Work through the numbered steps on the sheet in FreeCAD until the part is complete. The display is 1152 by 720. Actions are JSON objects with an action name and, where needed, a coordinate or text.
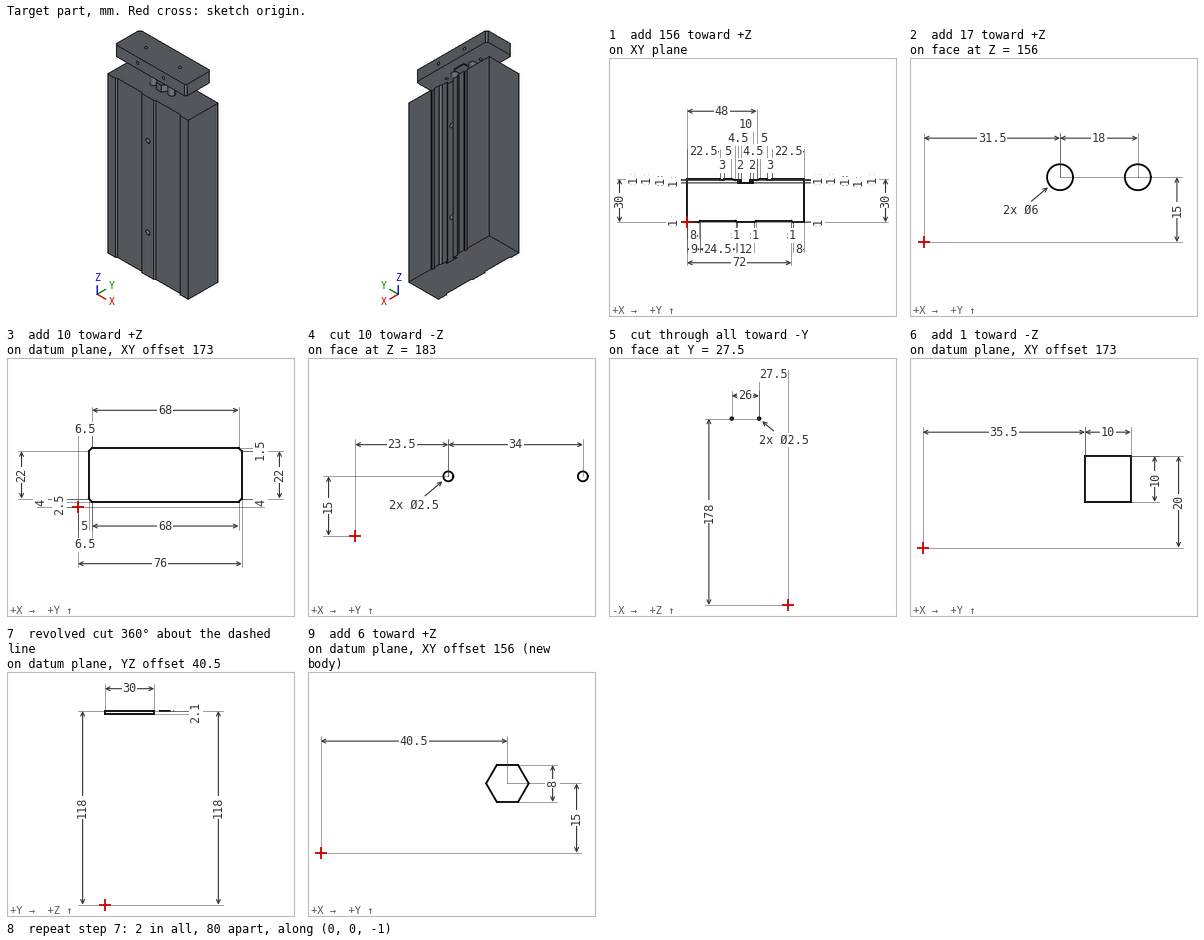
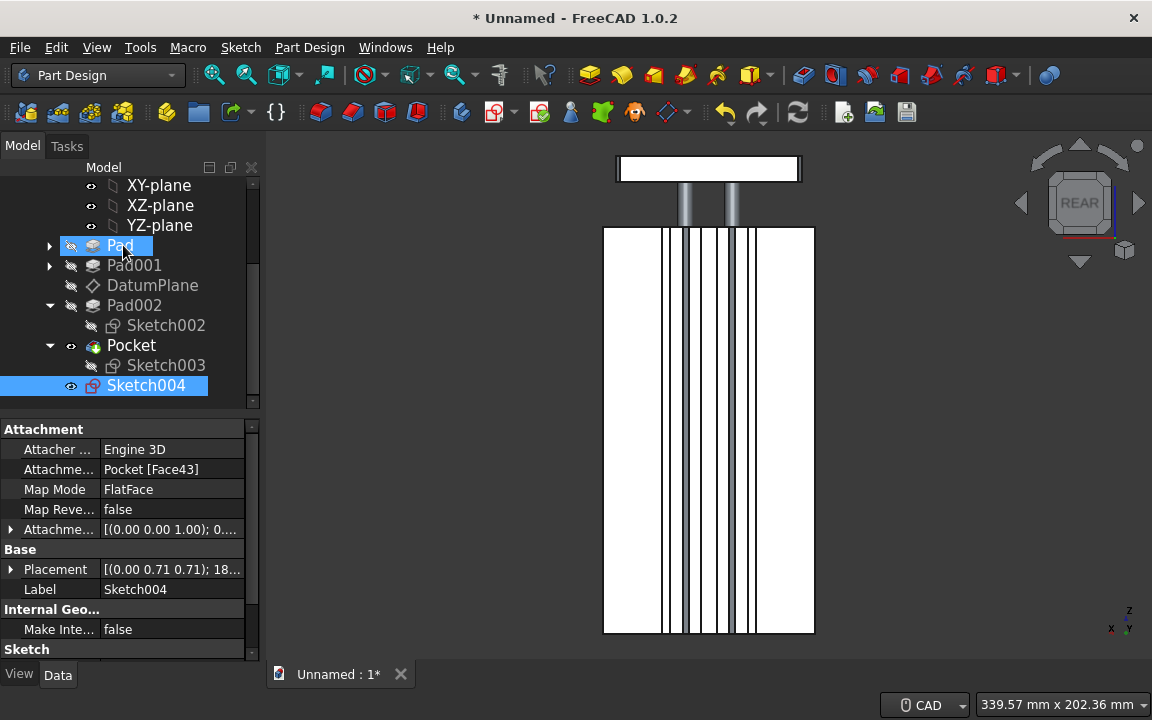
{"action": "left_click", "coordinate": [804, 76]}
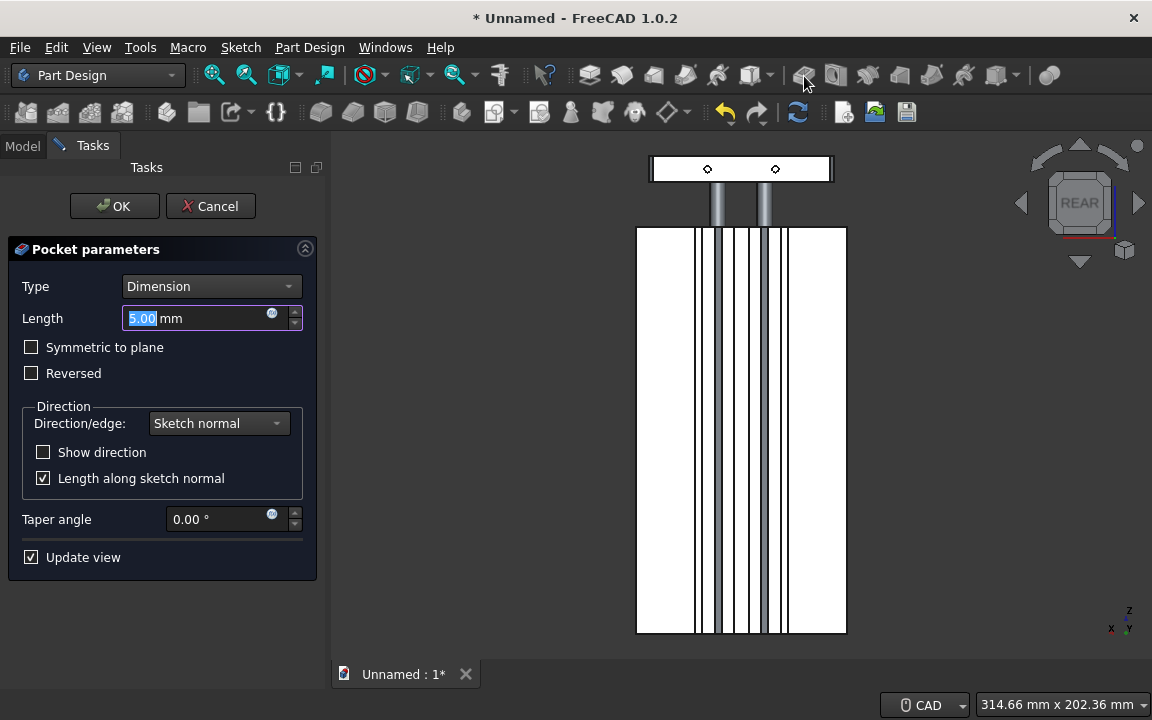
{"action": "left_click", "coordinate": [212, 286]}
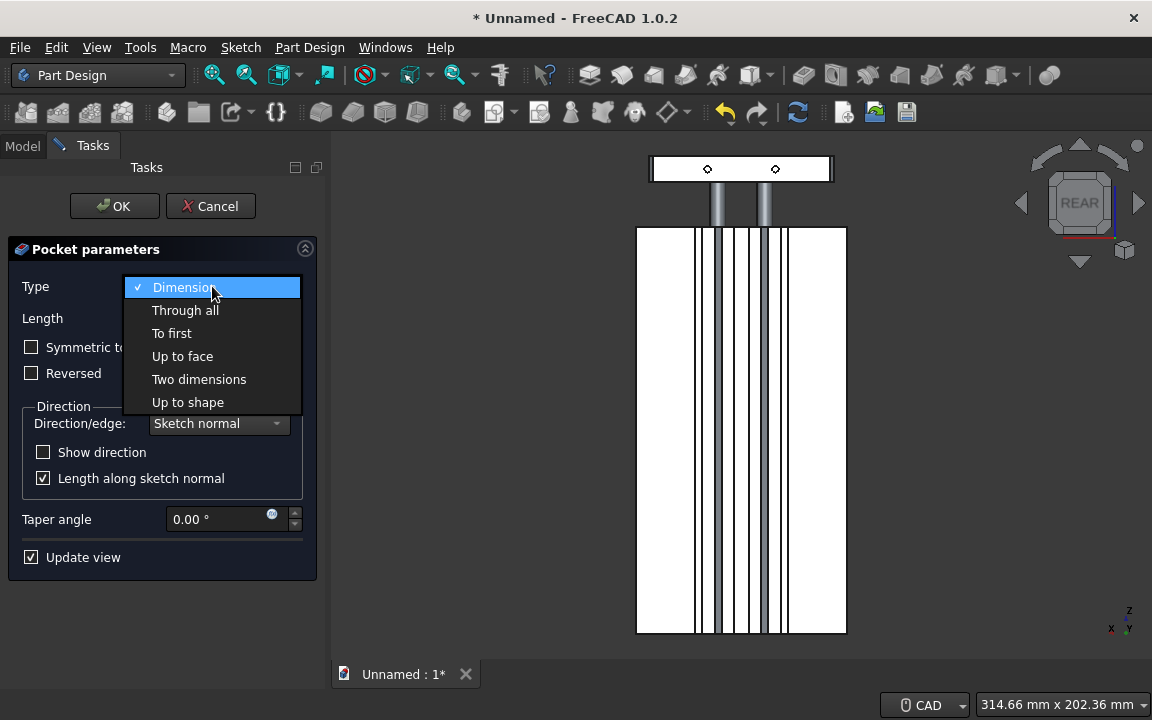
{"action": "left_click", "coordinate": [212, 310]}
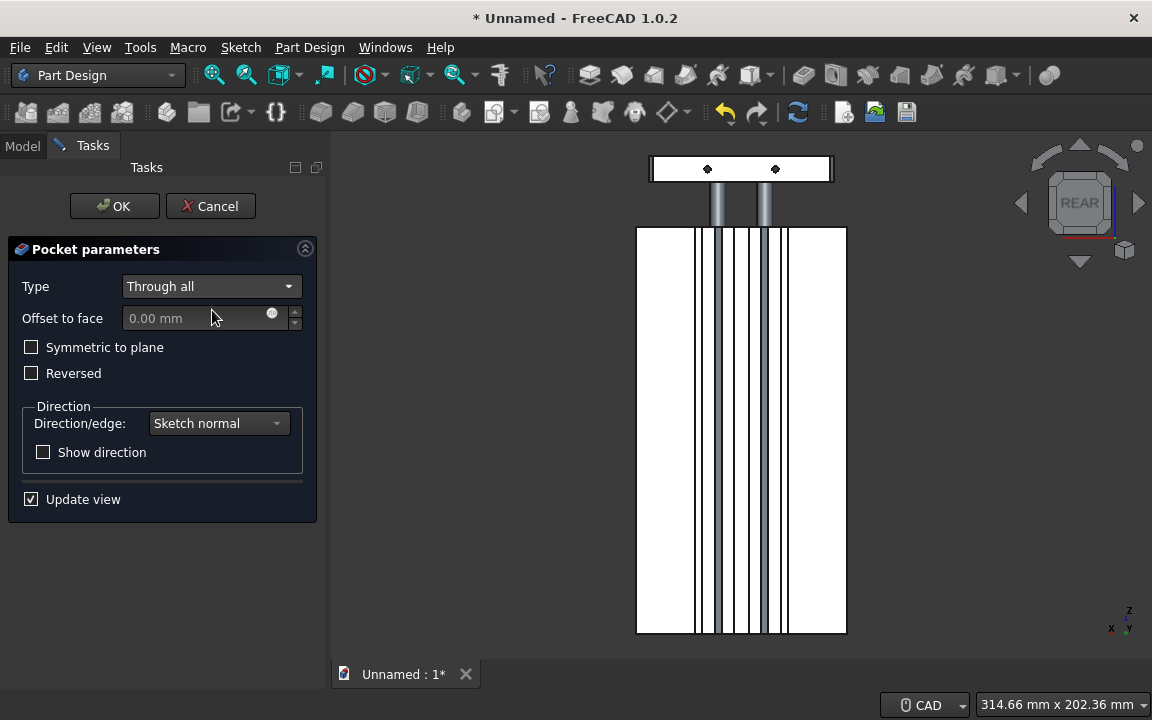
{"action": "left_click", "coordinate": [115, 206]}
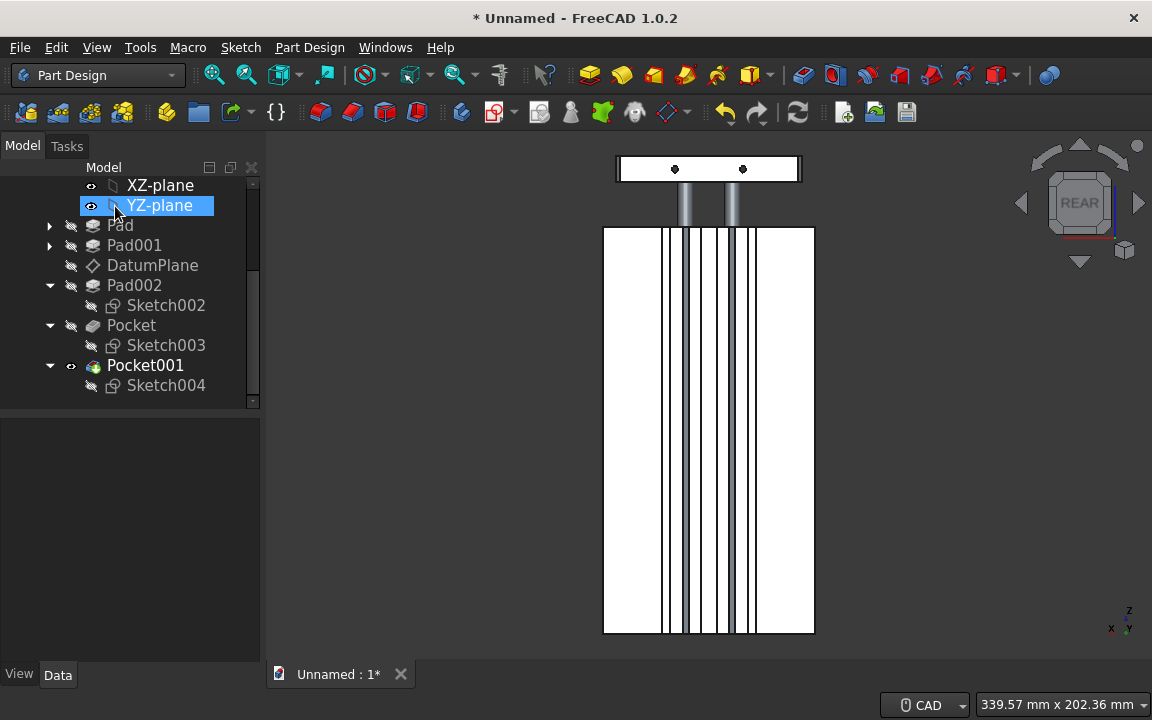
{"action": "scroll", "coordinate": [160, 281], "scroll_direction": "down", "scroll_amount": 3}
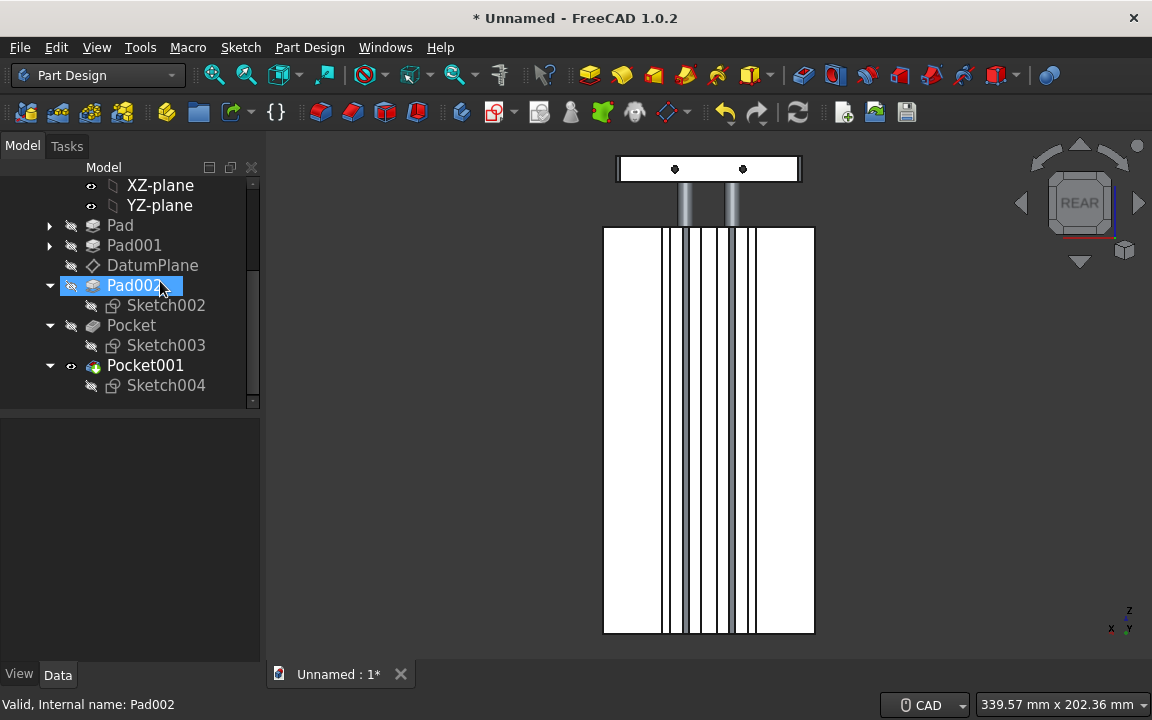
{"action": "scroll", "coordinate": [160, 281], "scroll_direction": "up", "scroll_amount": 15}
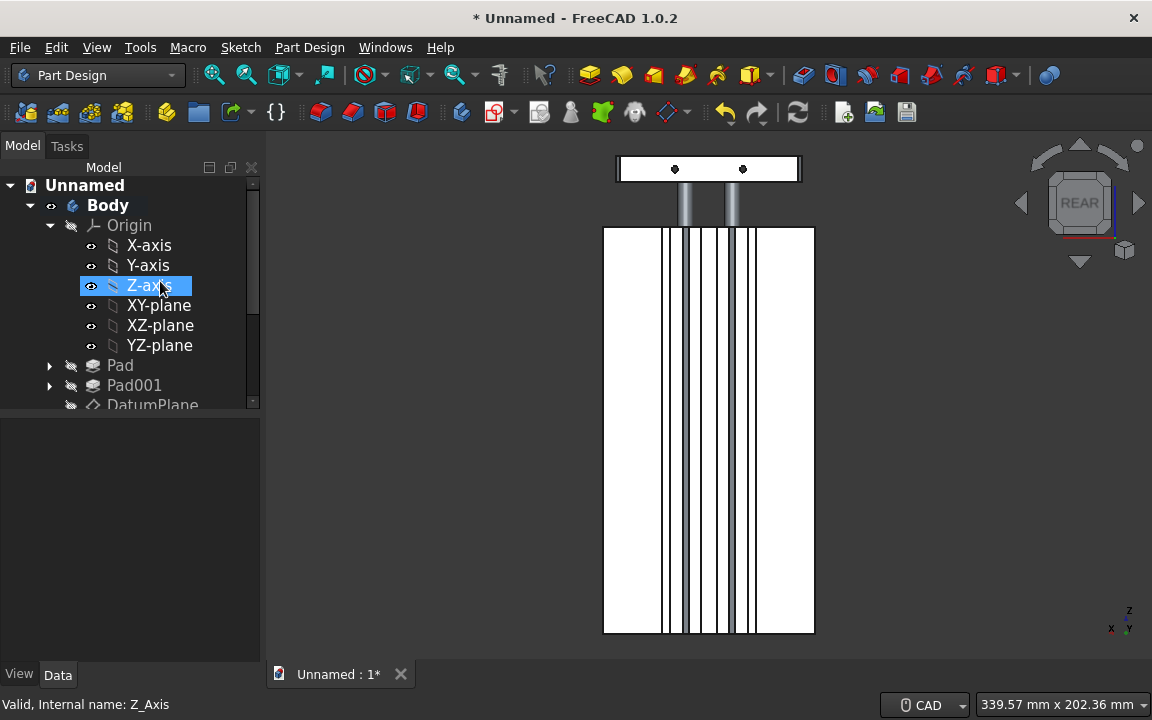
{"action": "left_click", "coordinate": [136, 306]}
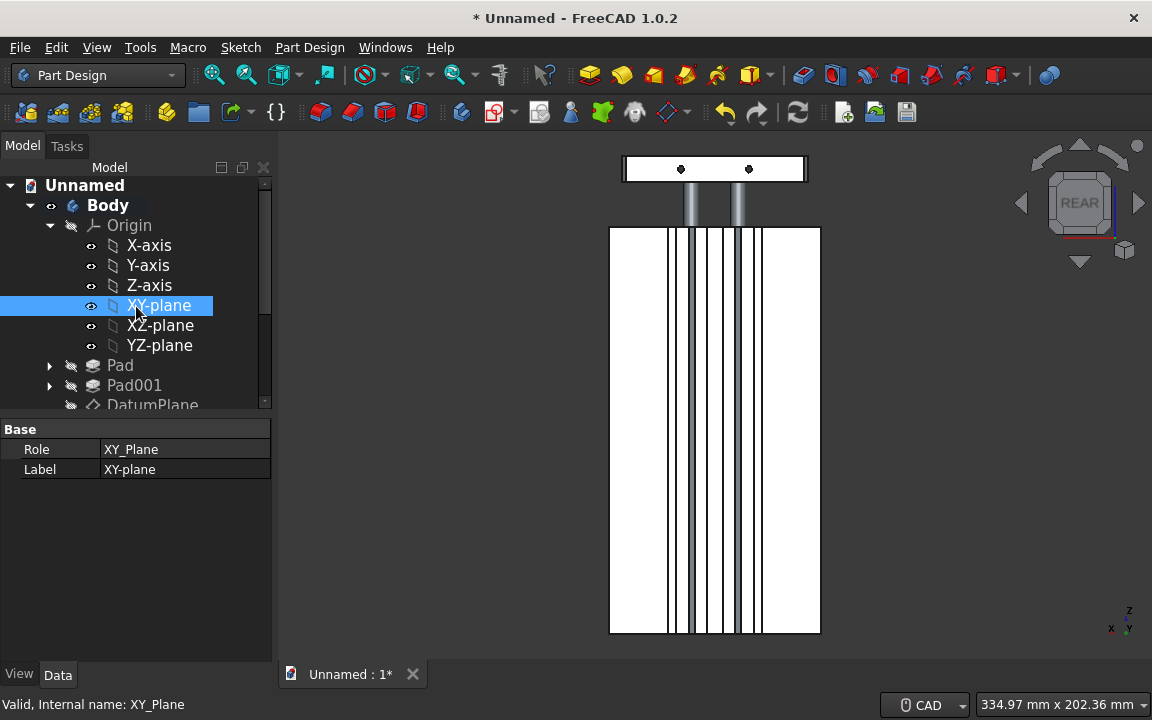
{"action": "left_click", "coordinate": [668, 112]}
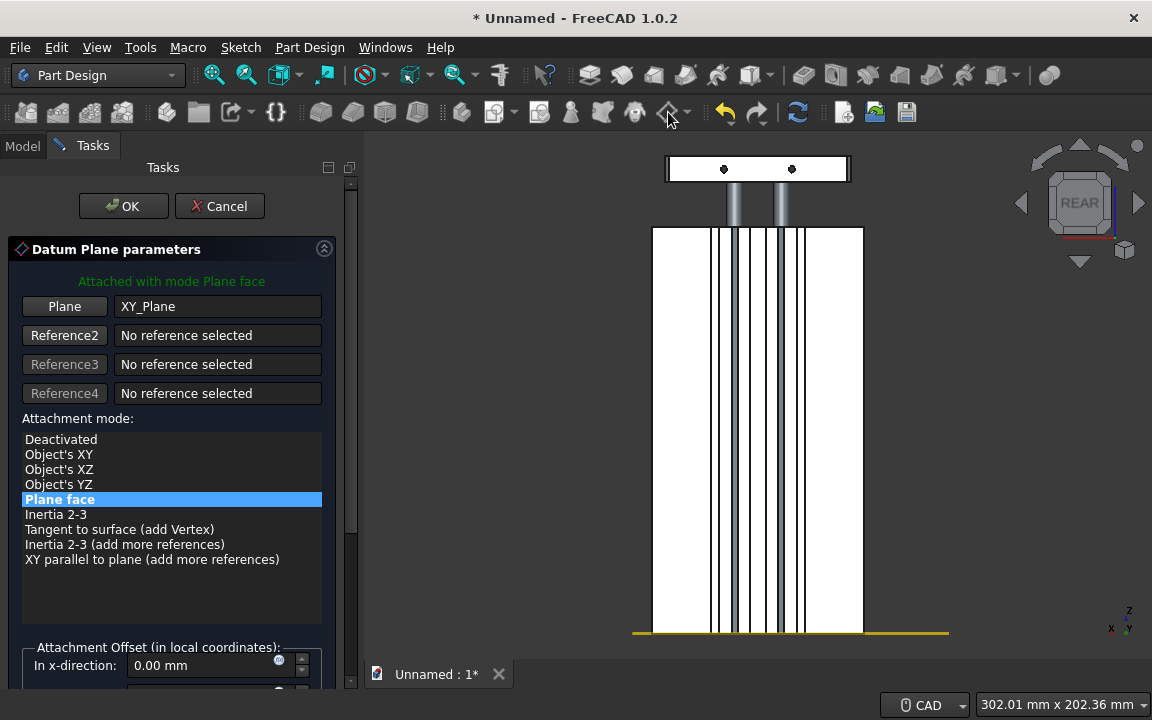
{"action": "scroll", "coordinate": [351, 432], "scroll_direction": "down", "scroll_amount": 2}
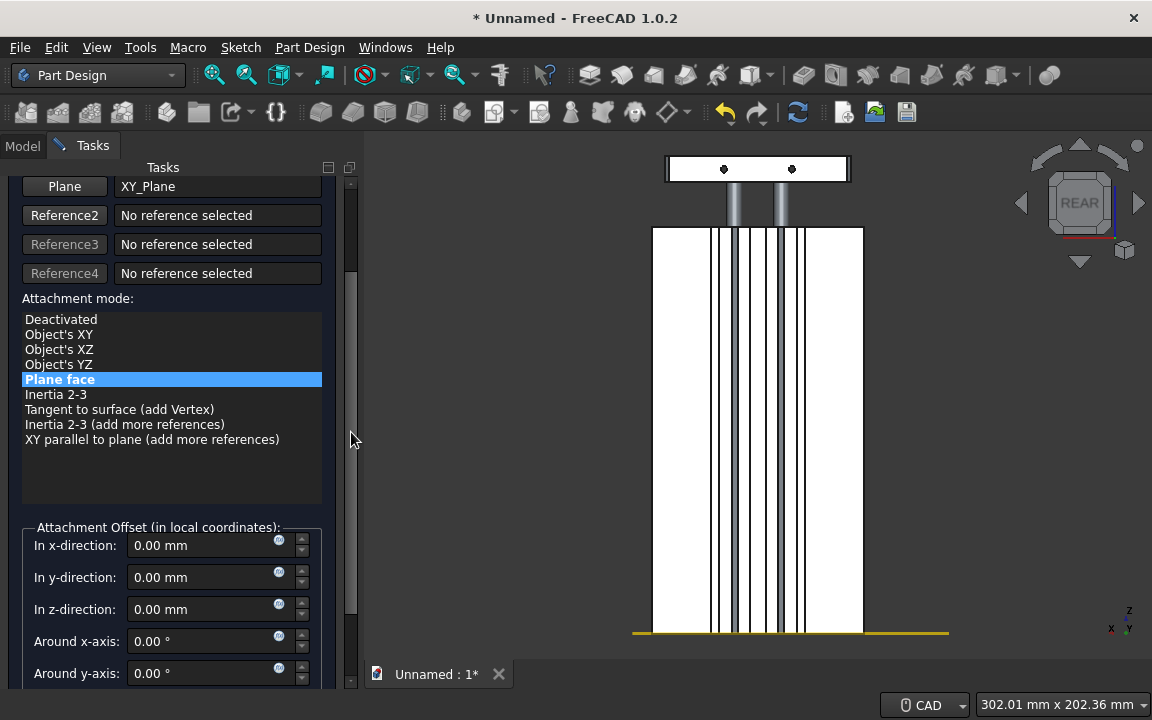
{"action": "triple_click", "coordinate": [210, 609]}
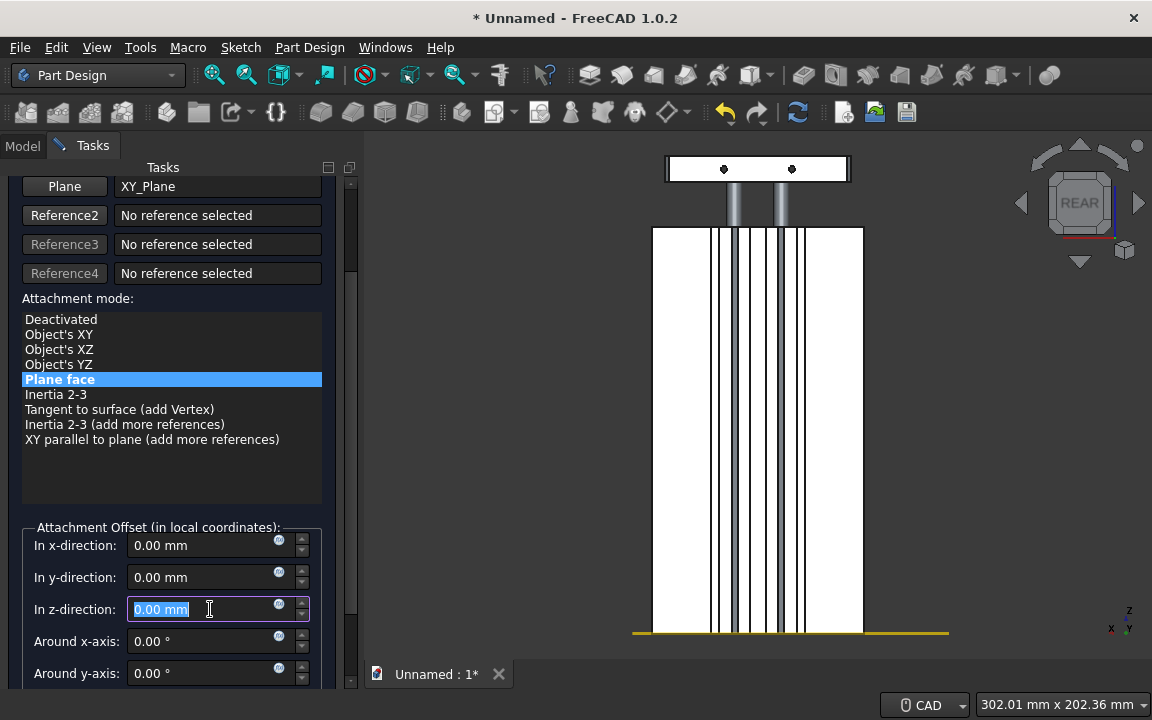
{"action": "type", "text": "173"}
{"action": "key", "text": "Tab"}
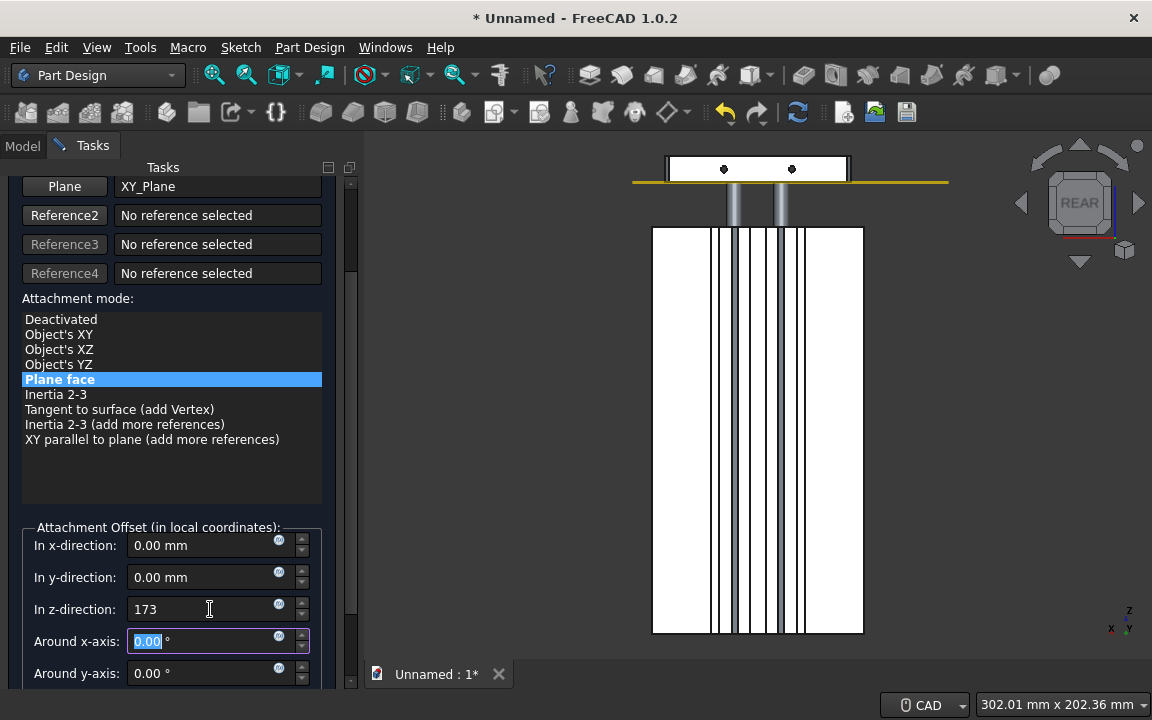
{"action": "scroll", "coordinate": [351, 432], "scroll_direction": "up", "scroll_amount": 3}